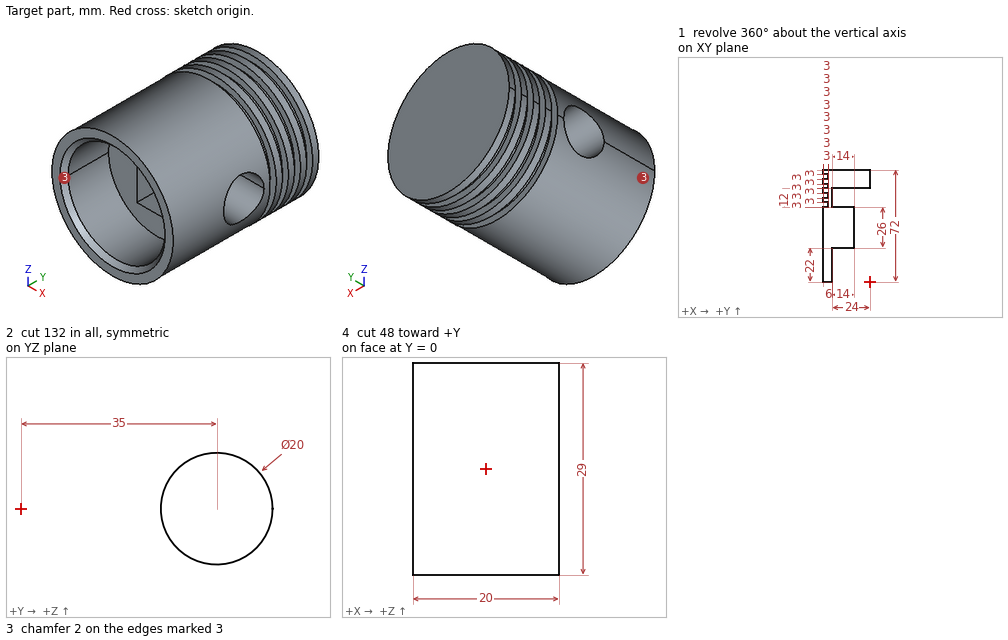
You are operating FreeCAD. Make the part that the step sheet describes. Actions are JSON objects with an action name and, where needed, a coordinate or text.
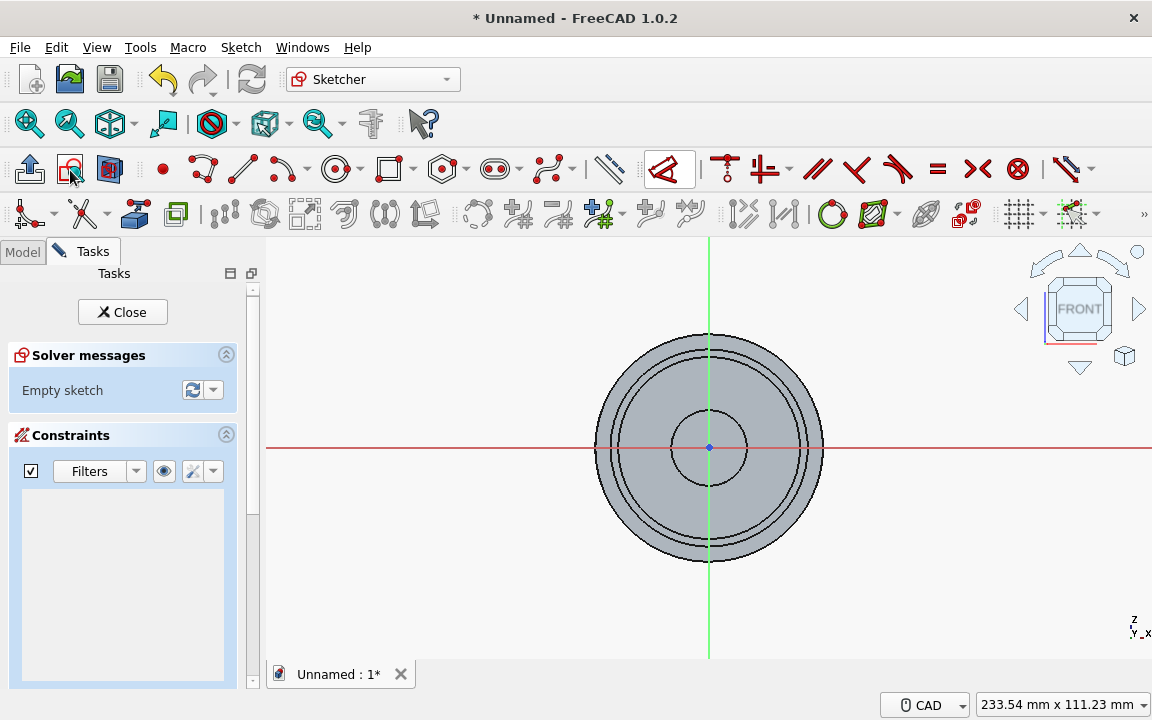
{"action": "scroll", "coordinate": [765, 448], "scroll_direction": "up", "scroll_amount": 4}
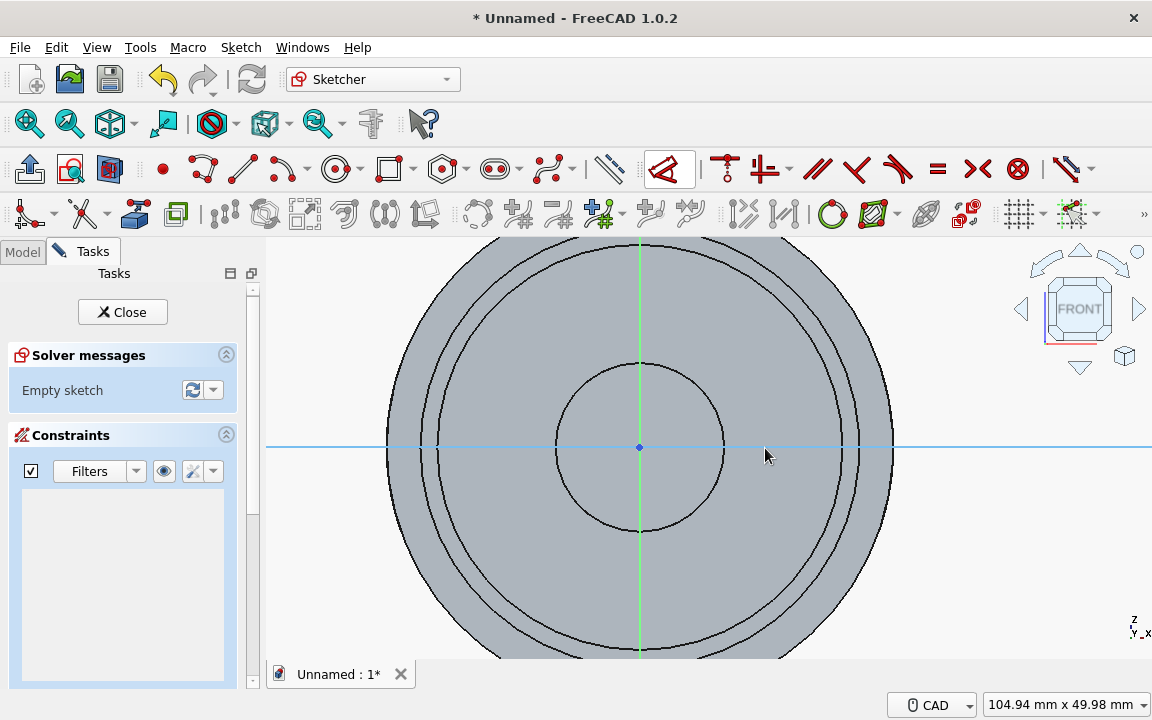
{"action": "left_click", "coordinate": [416, 170]}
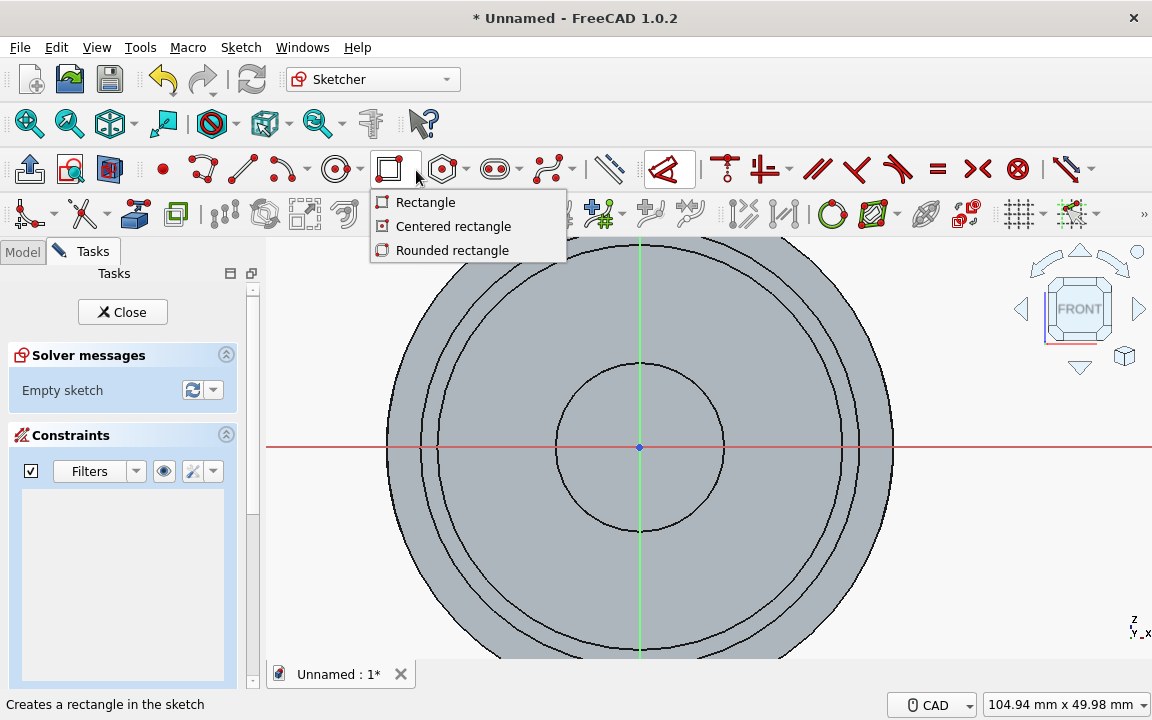
{"action": "left_click", "coordinate": [468, 226]}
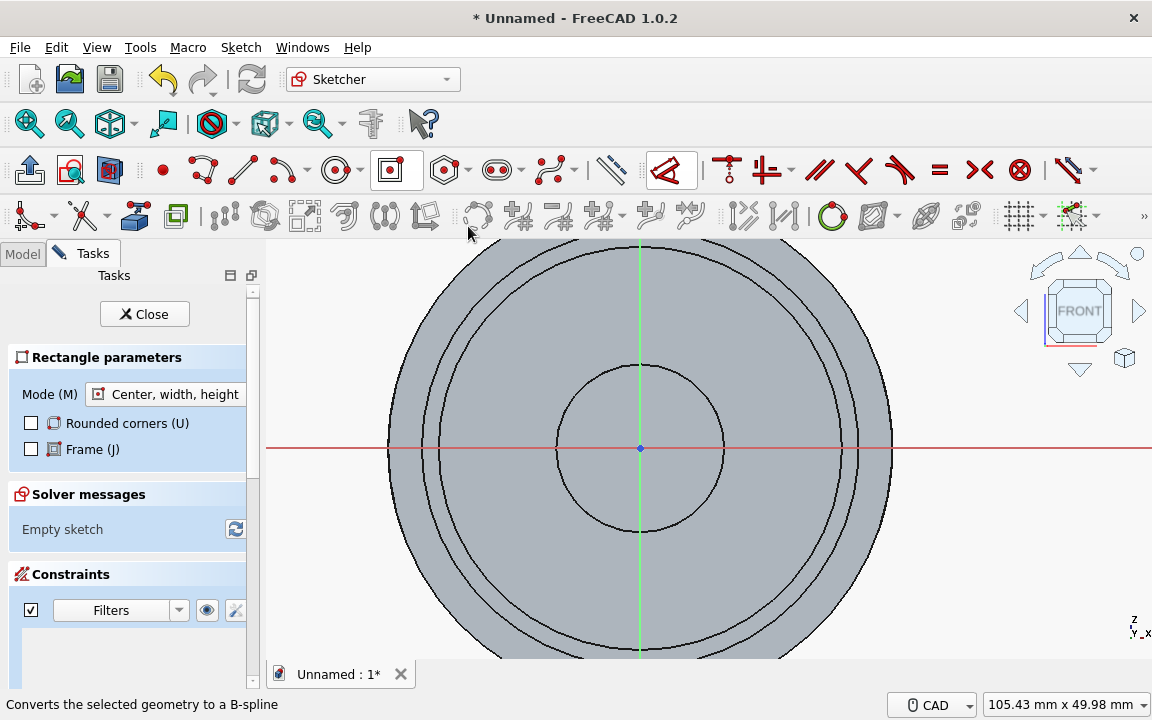
{"action": "left_click", "coordinate": [640, 448]}
{"action": "mouse_move", "coordinate": [724, 327]}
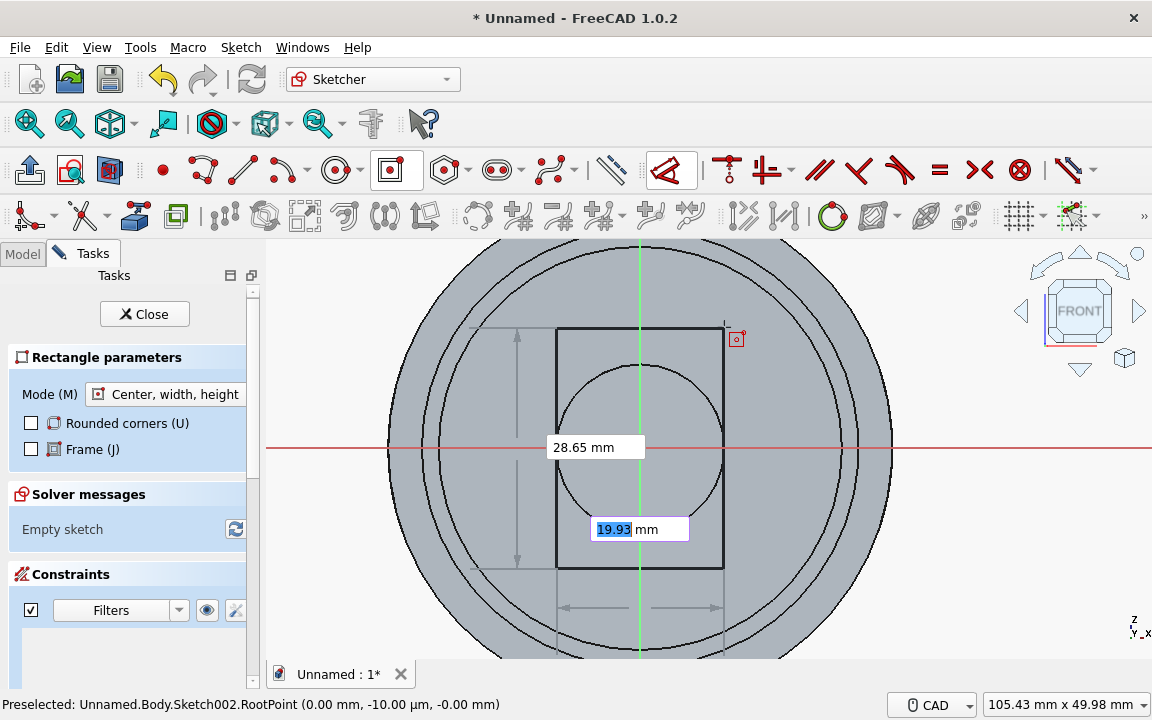
{"action": "type", "text": "20"}
{"action": "key", "text": "Tab"}
{"action": "type", "text": "29"}
{"action": "key", "text": "Return"}
{"action": "key", "text": "Escape"}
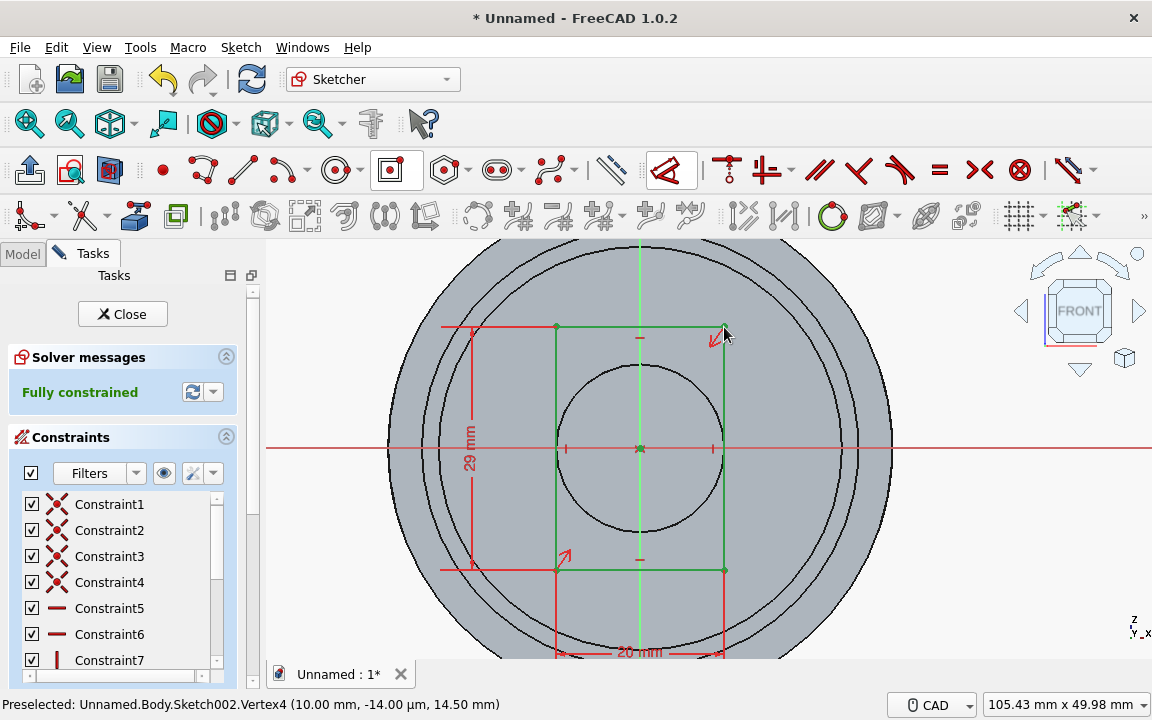
{"action": "left_click", "coordinate": [123, 314]}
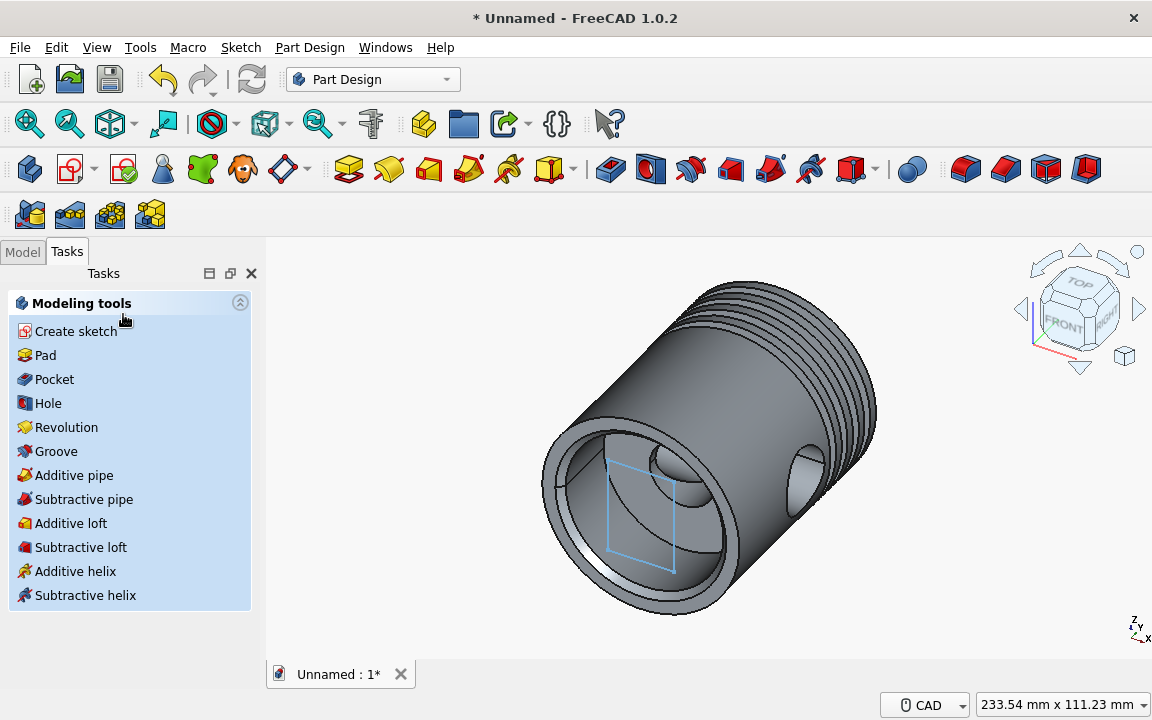
{"action": "left_click", "coordinate": [612, 170]}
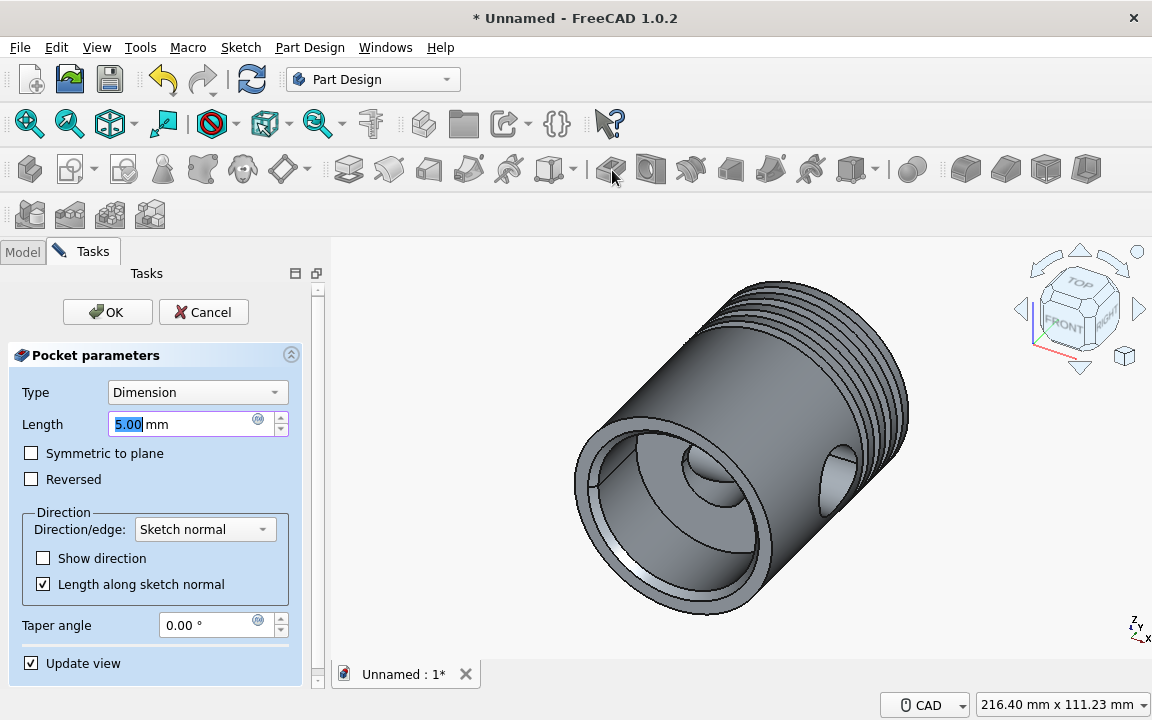
{"action": "type", "text": "48"}
{"action": "key", "text": "Tab"}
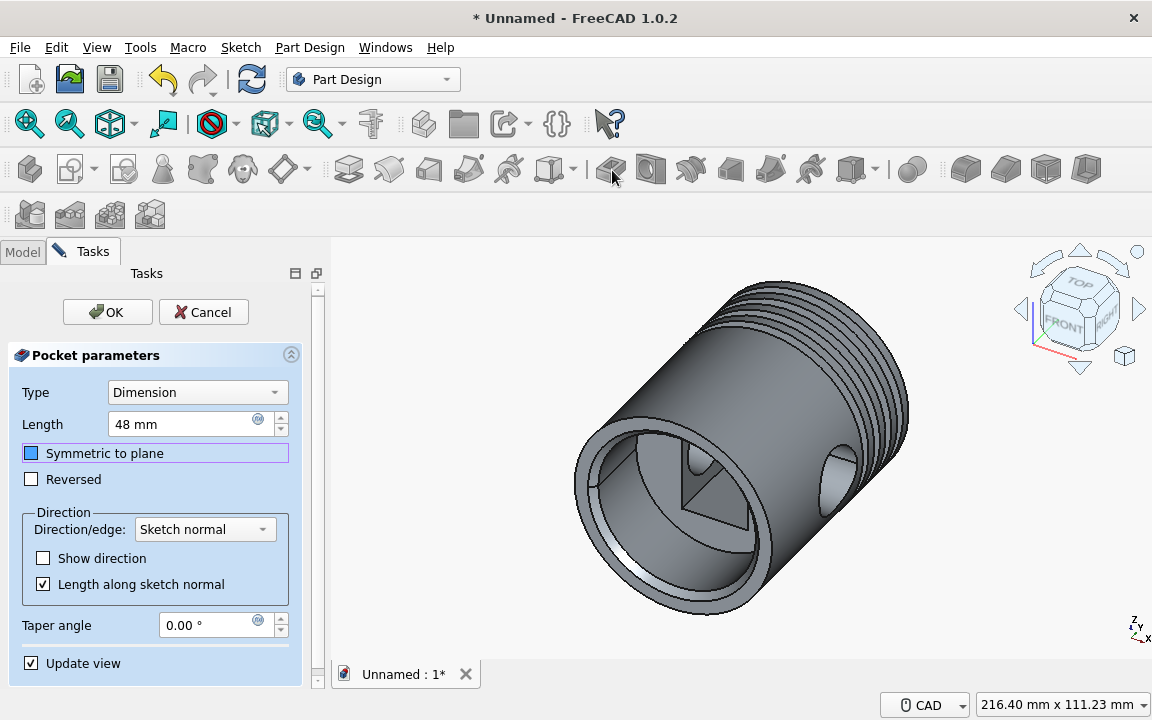
{"action": "left_click", "coordinate": [108, 312]}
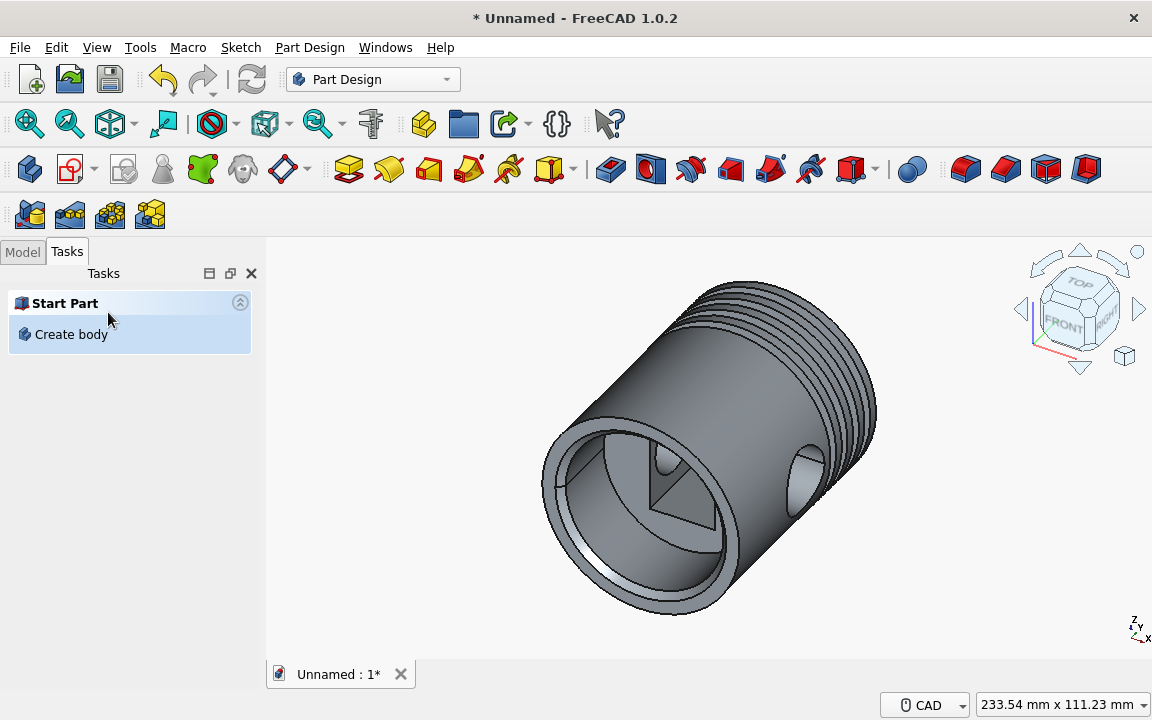
{"action": "key", "text": "0"}